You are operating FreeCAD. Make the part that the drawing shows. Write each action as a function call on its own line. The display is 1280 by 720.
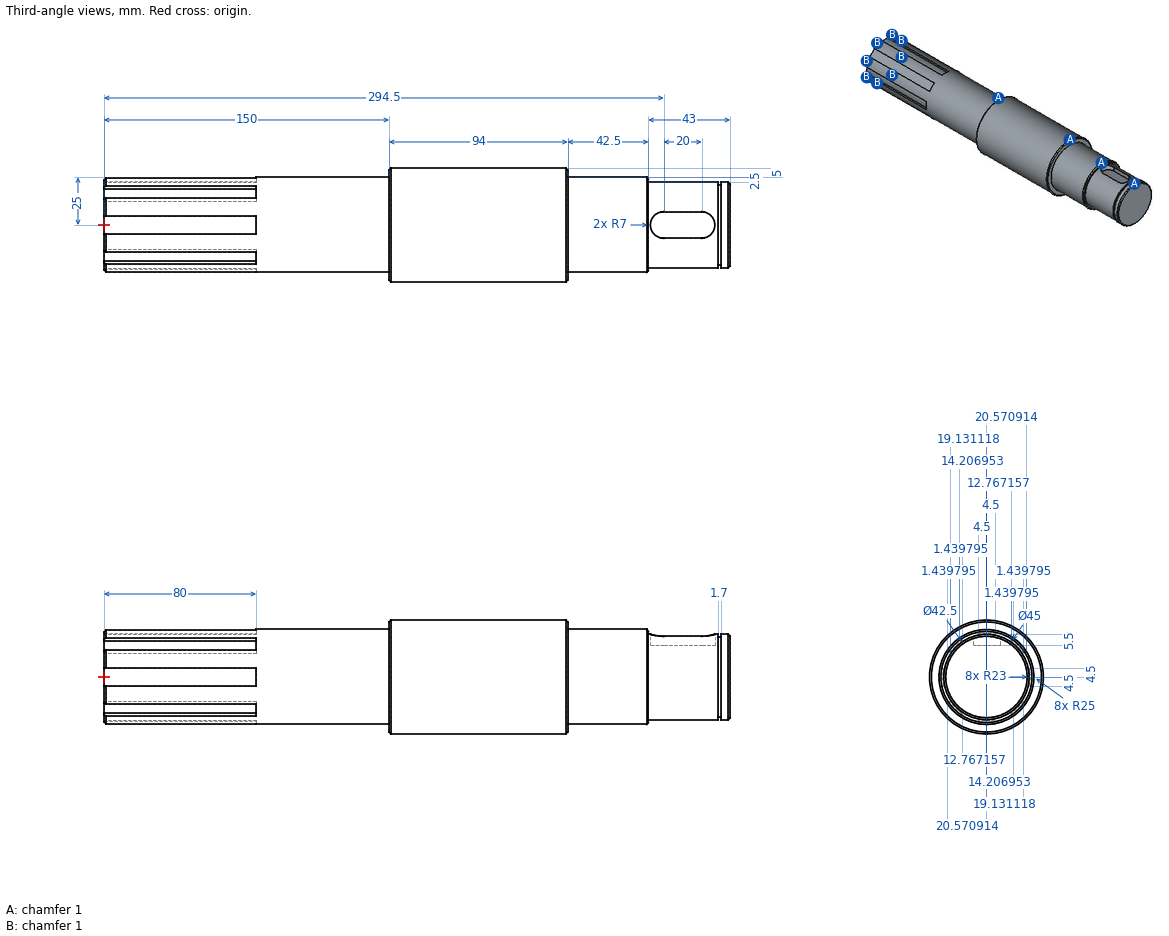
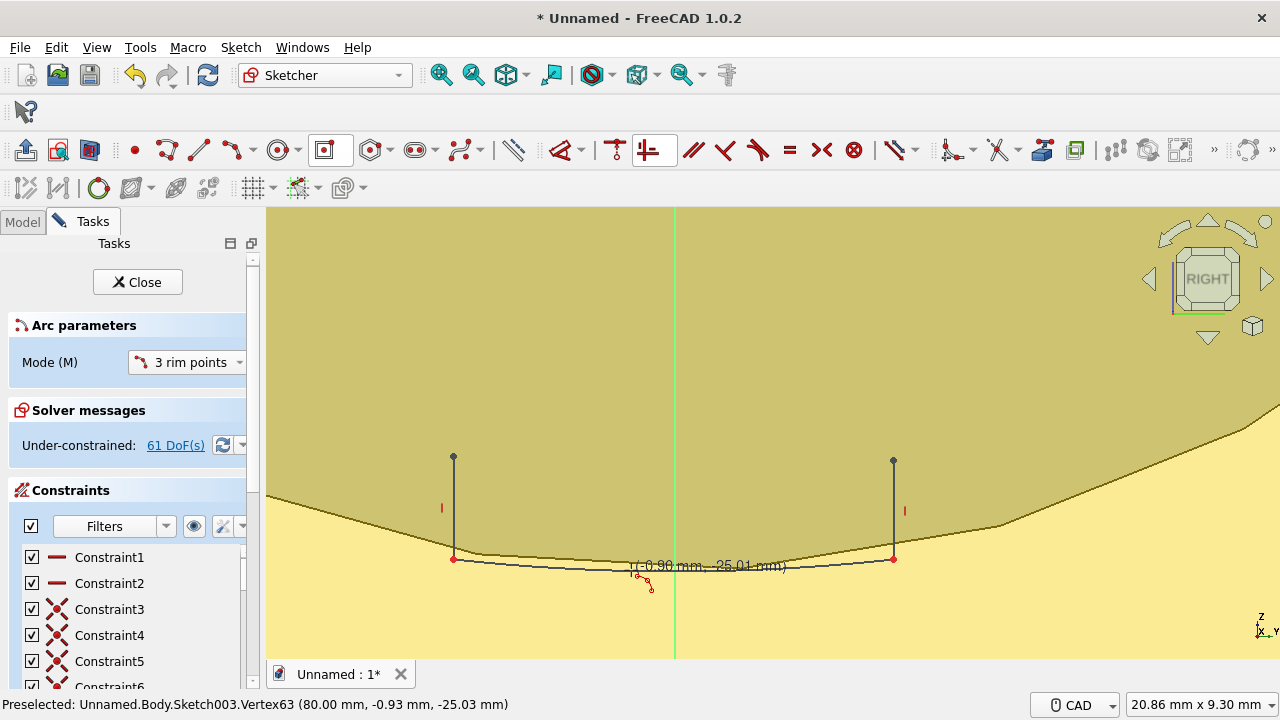
scroll(708, 567, down, 11)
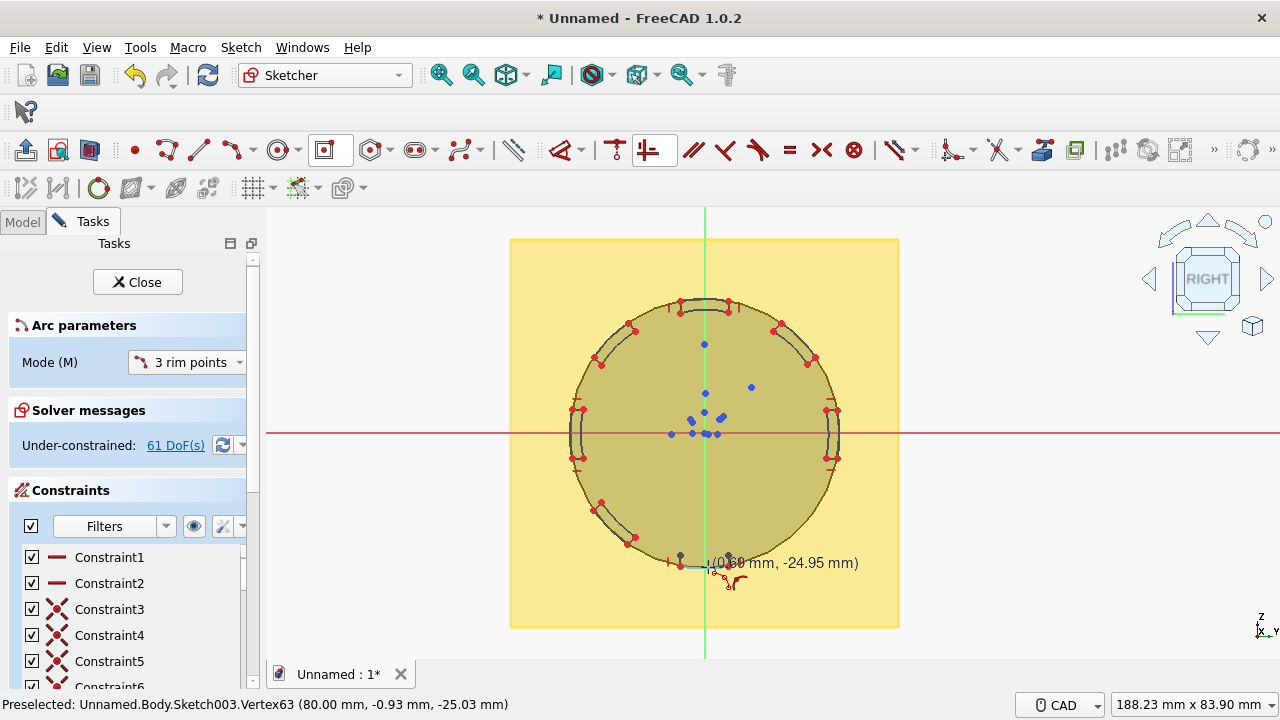
scroll(680, 555, up, 6)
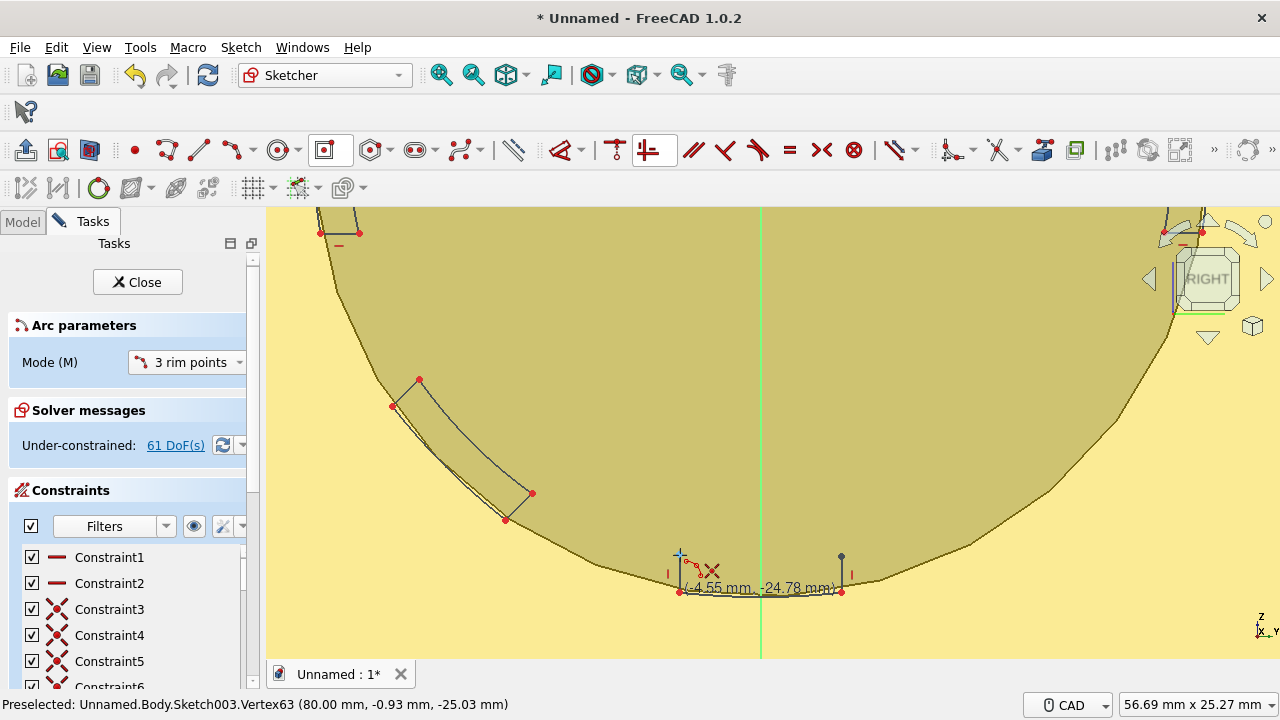
click(680, 555)
click(842, 556)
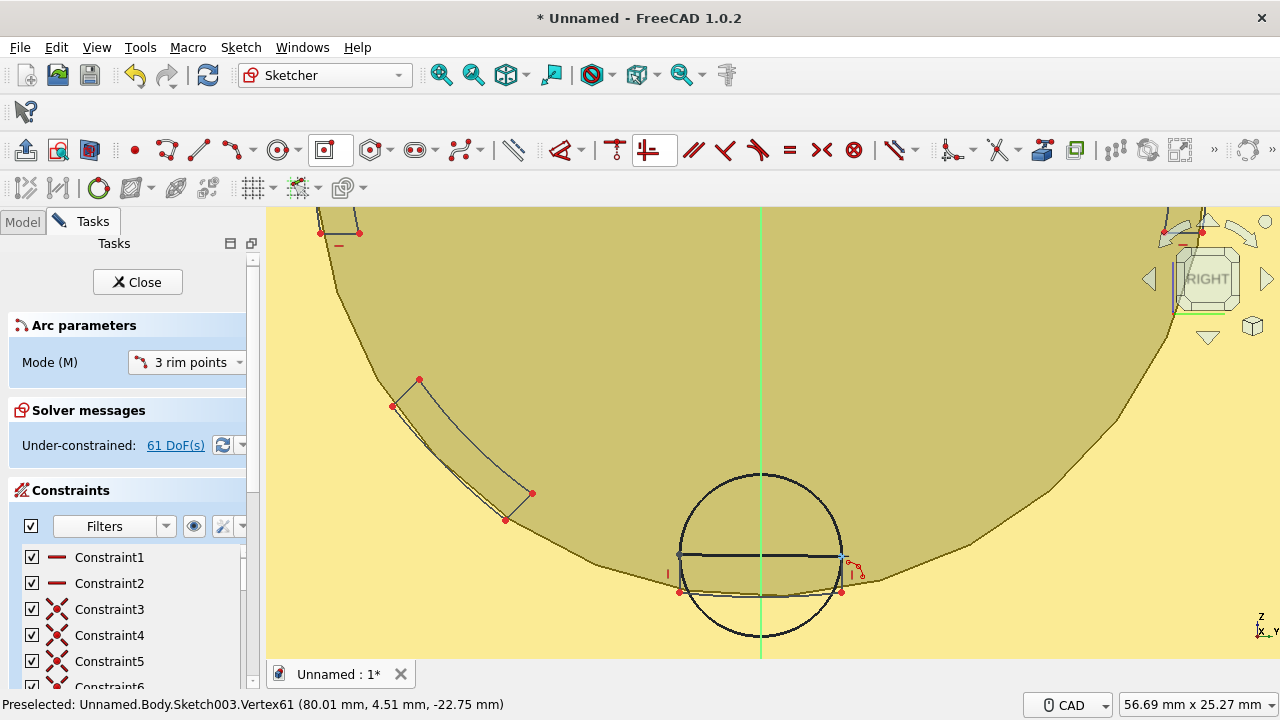
scroll(745, 561, up, 4)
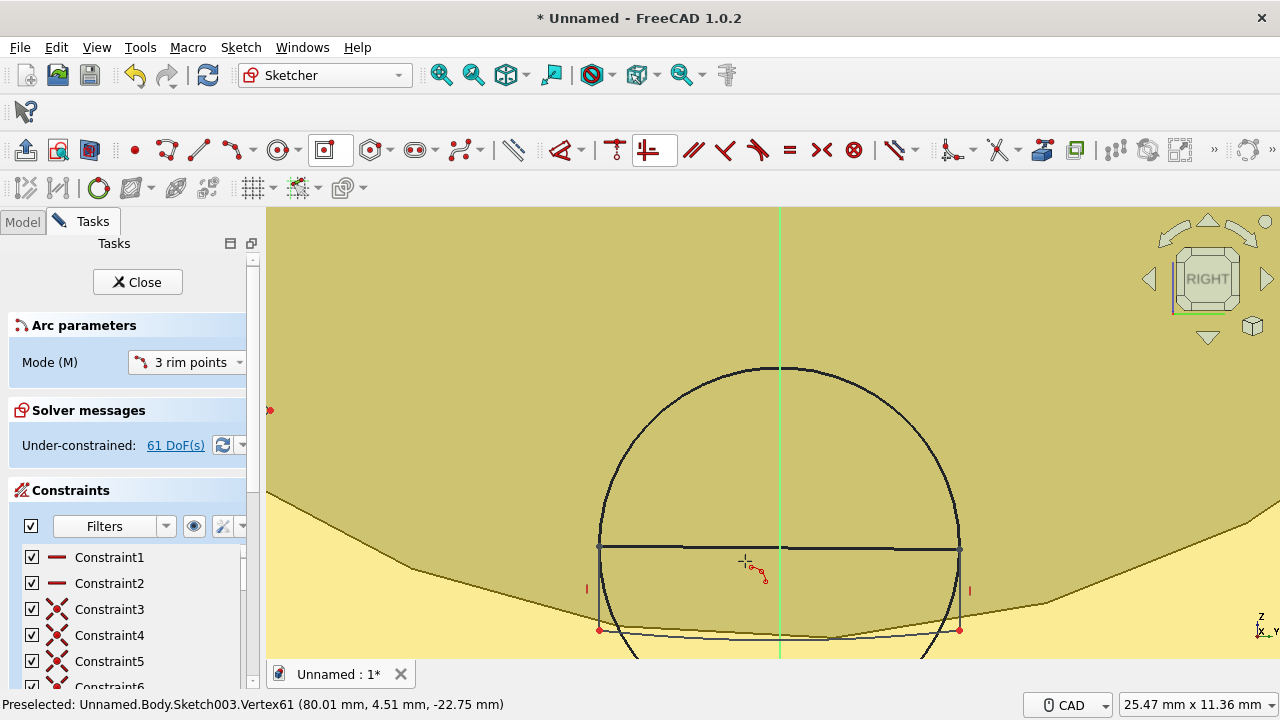
click(744, 559)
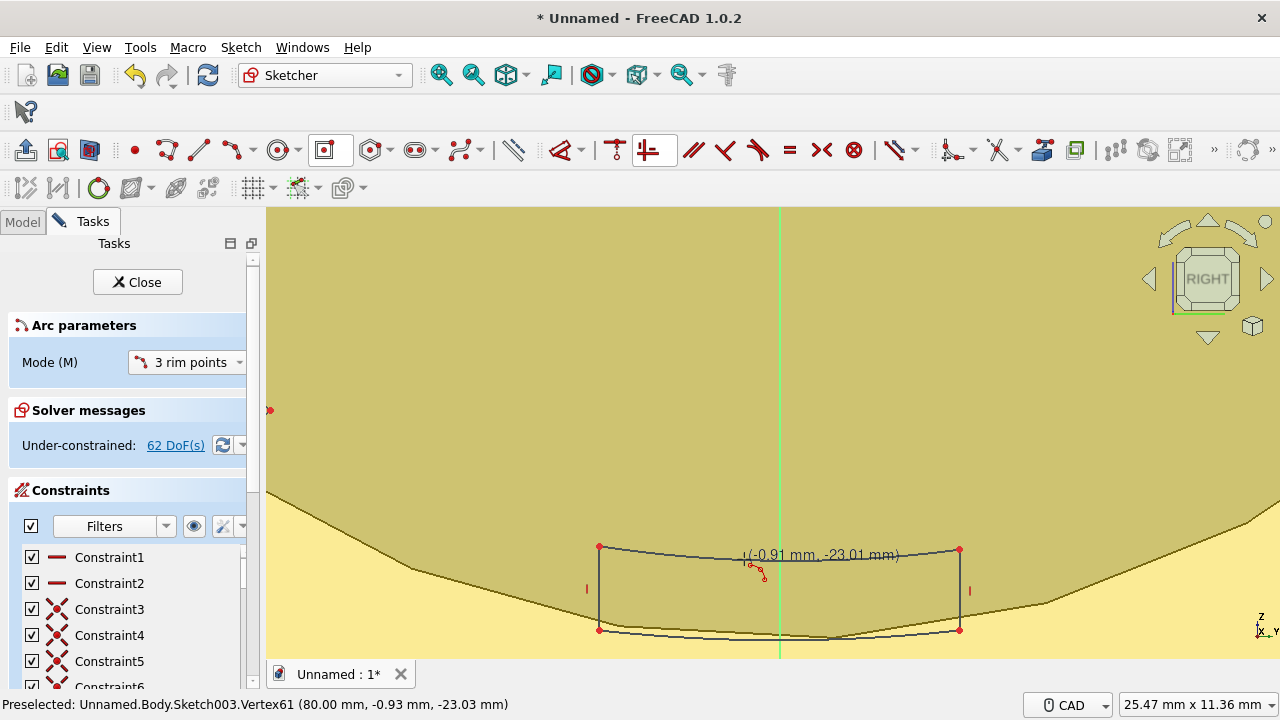
click(200, 150)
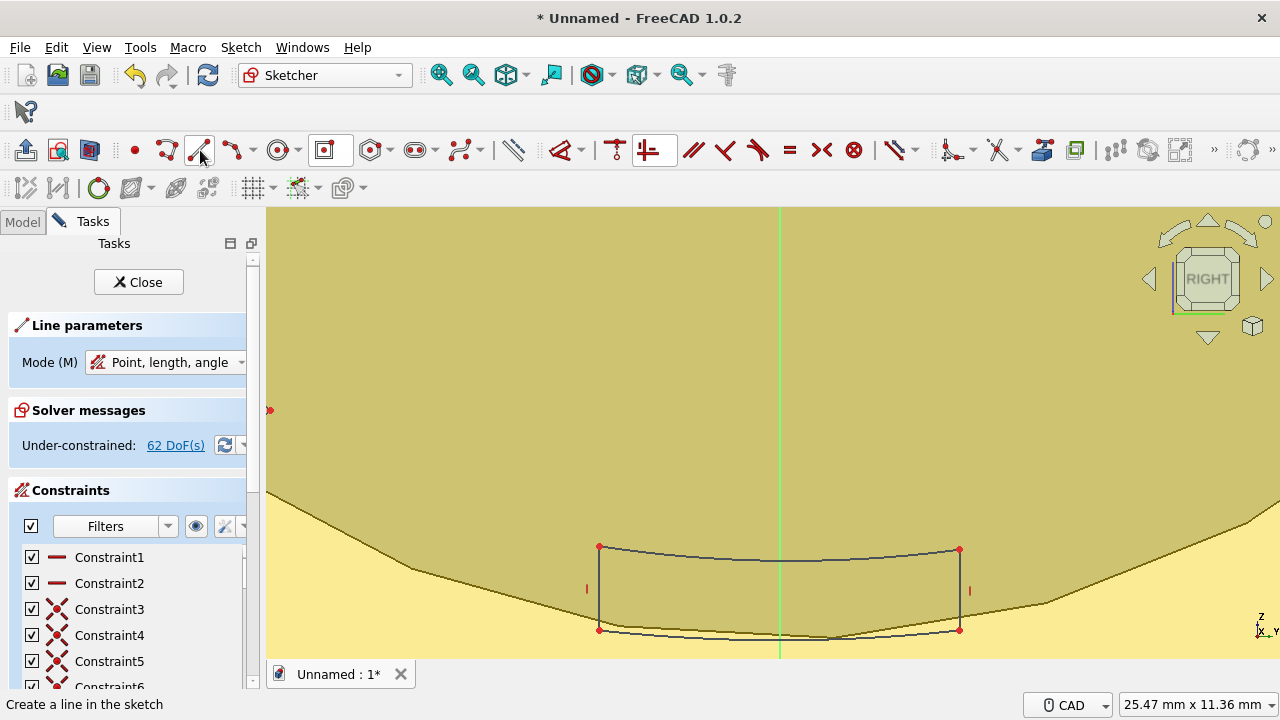
scroll(693, 556, down, 10)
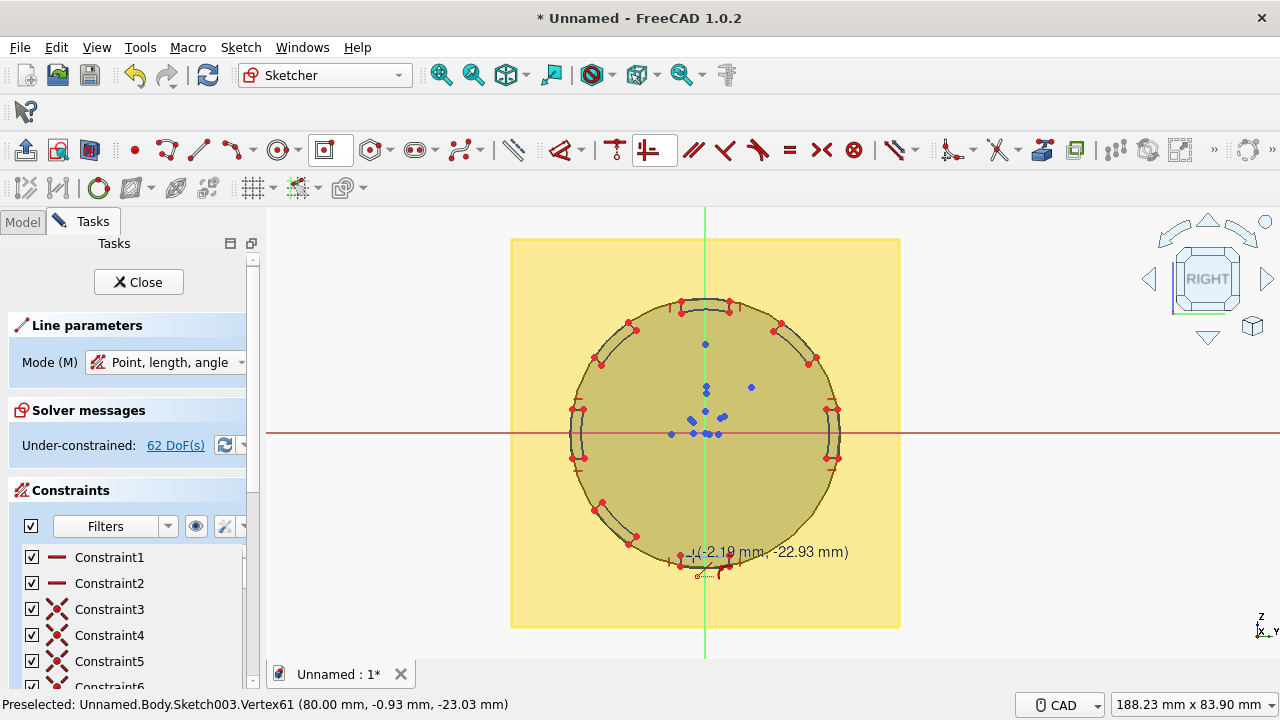
click(808, 502)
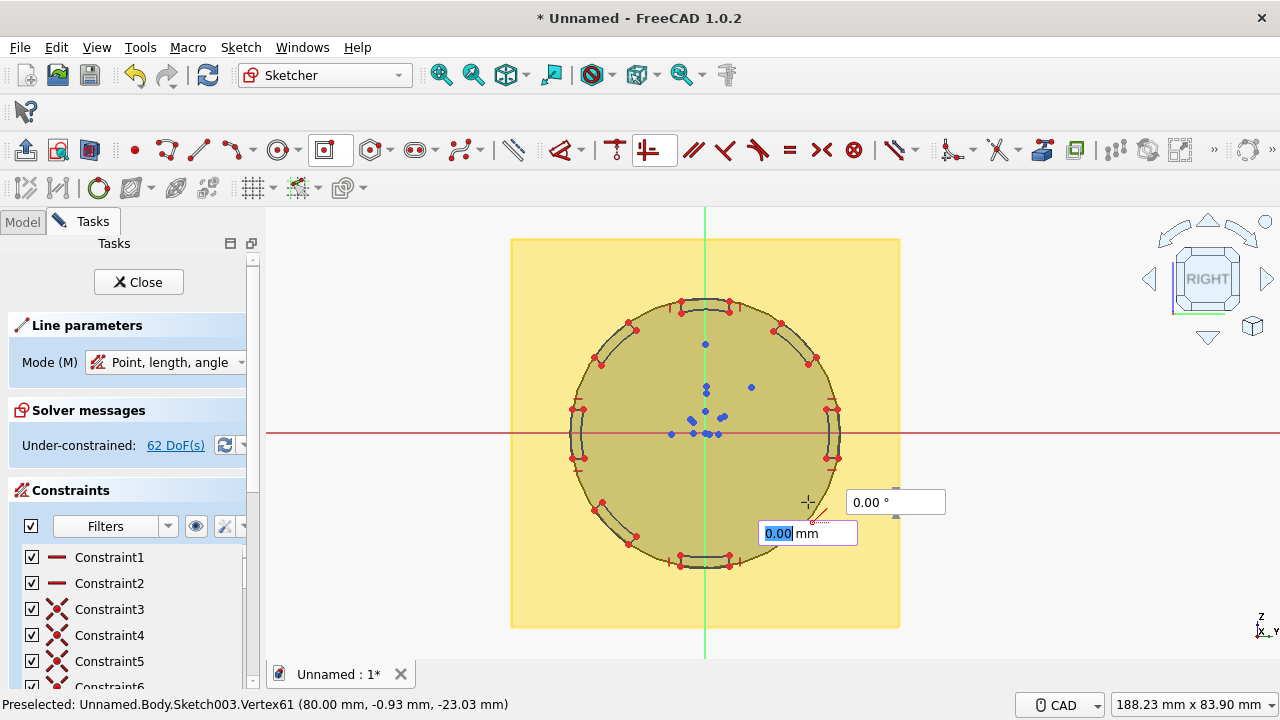
scroll(816, 510, up, 2)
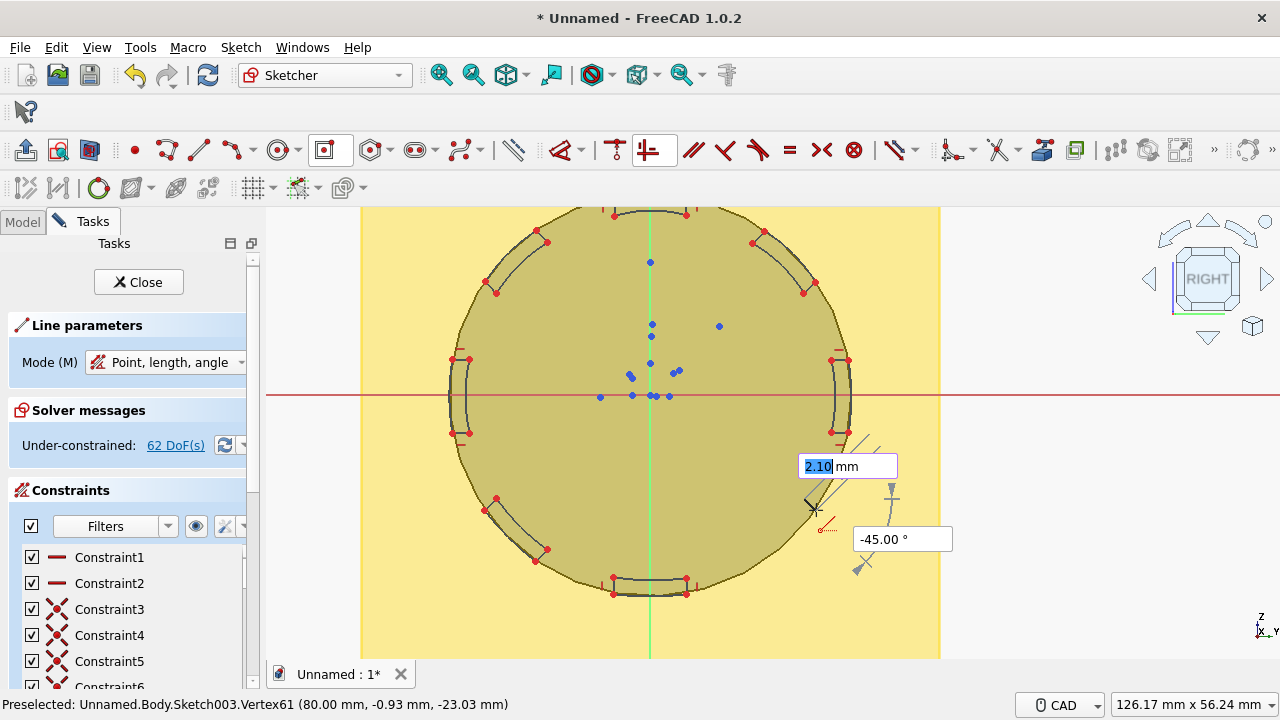
click(816, 509)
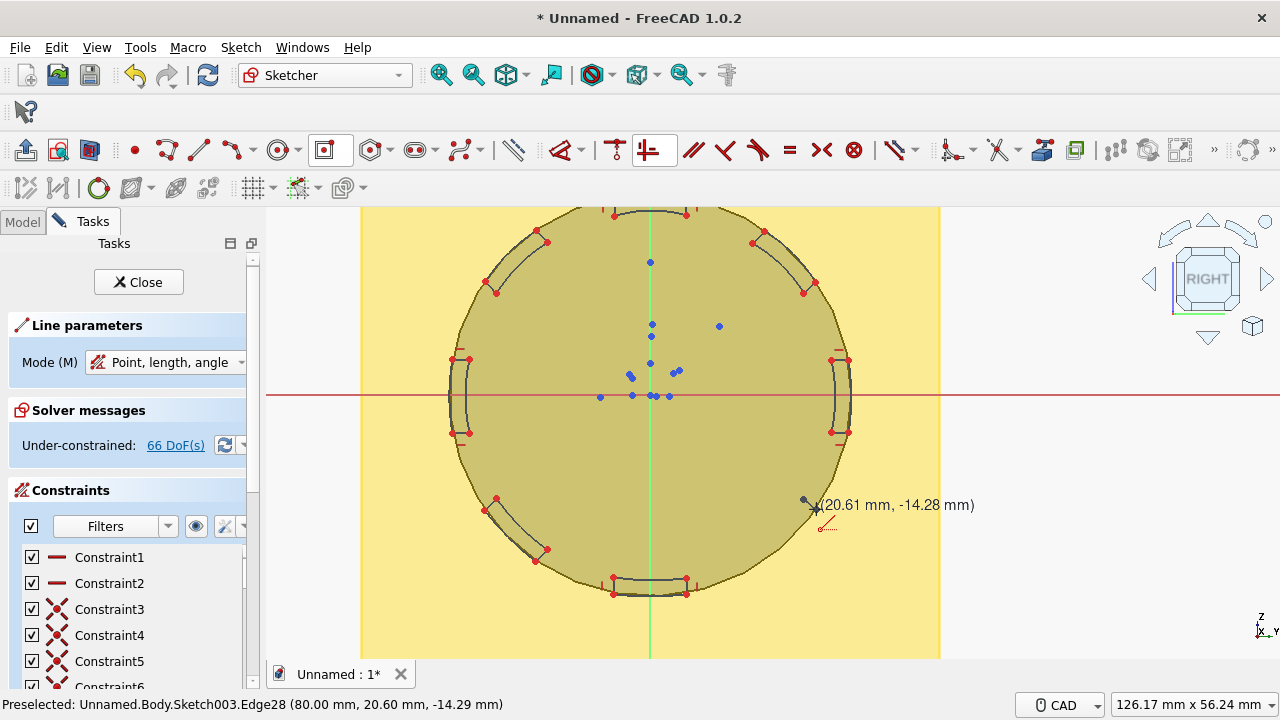
click(765, 561)
click(753, 549)